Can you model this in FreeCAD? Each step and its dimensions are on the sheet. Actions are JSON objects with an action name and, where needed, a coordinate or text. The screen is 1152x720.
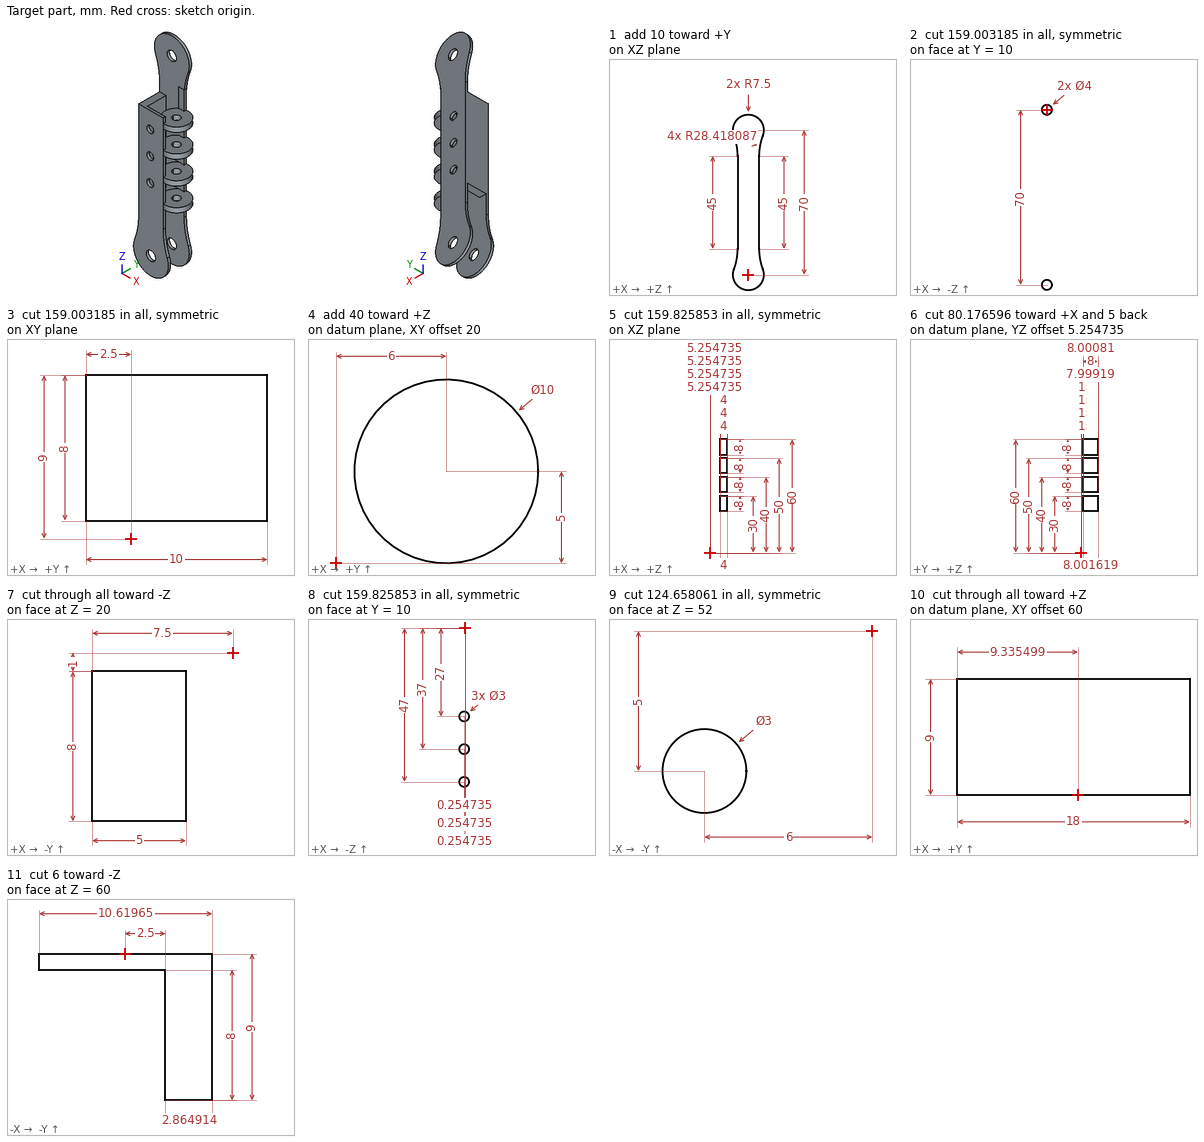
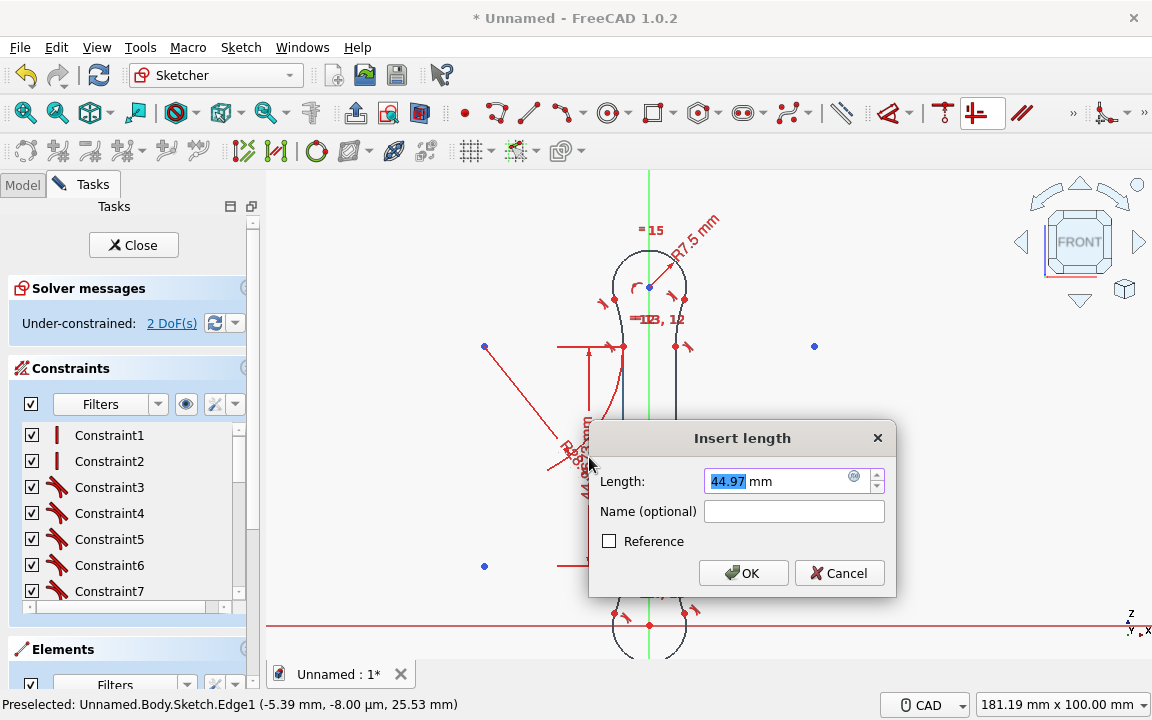
{"action": "type", "text": "45"}
{"action": "key", "text": "Return"}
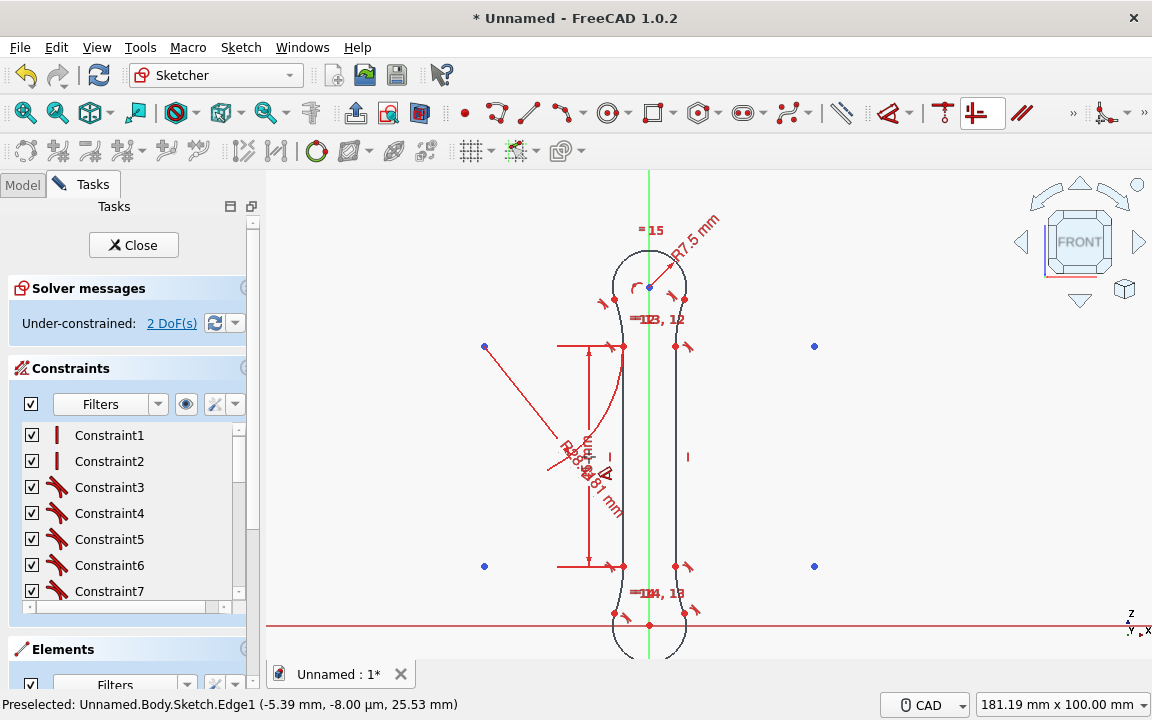
{"action": "left_click", "coordinate": [676, 412]}
{"action": "left_click", "coordinate": [710, 457]}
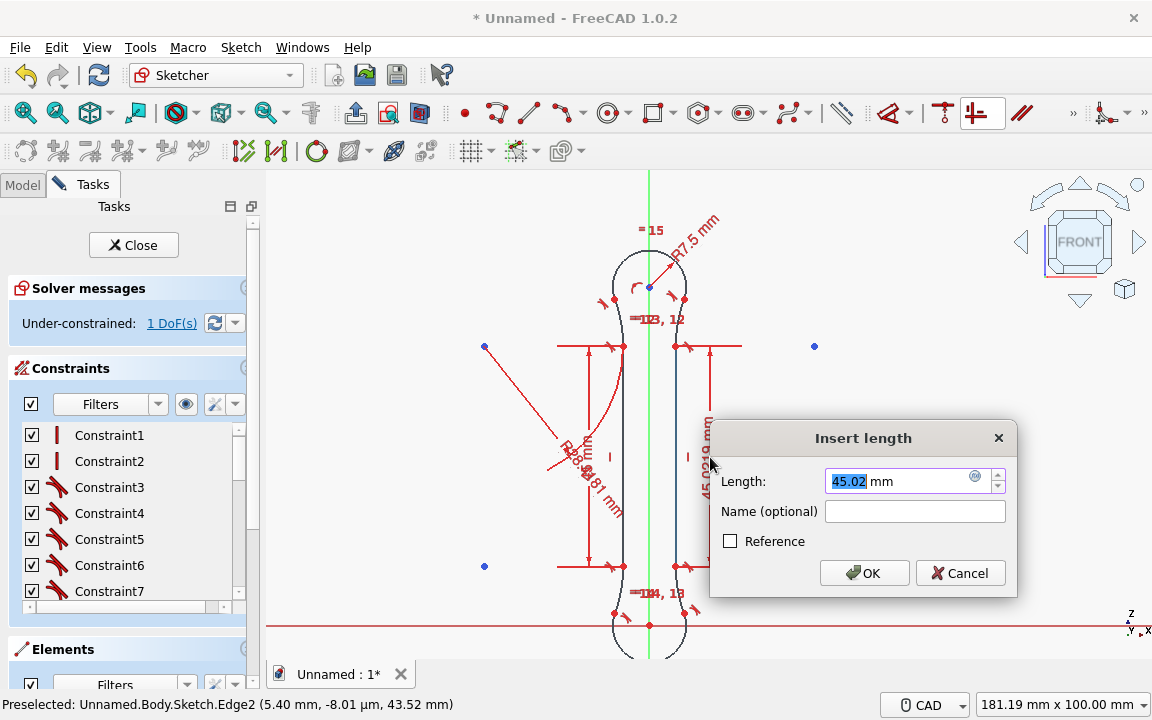
{"action": "type", "text": "45"}
{"action": "key", "text": "Return"}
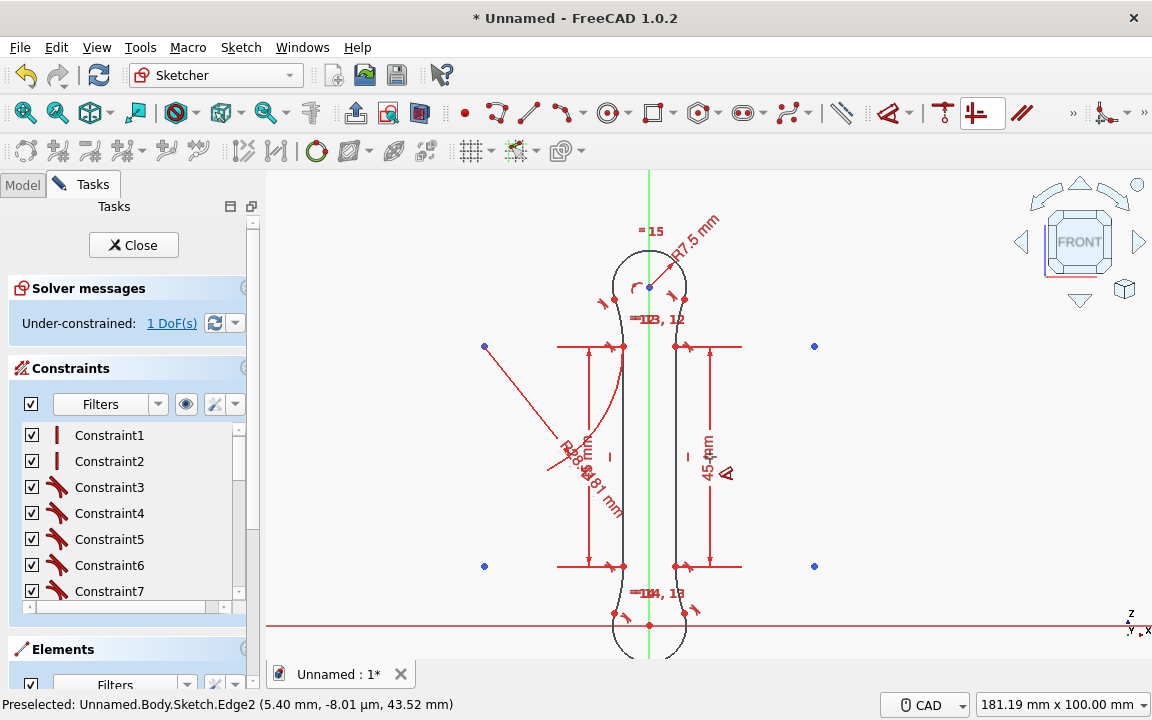
{"action": "left_click", "coordinate": [649, 287]}
{"action": "left_click", "coordinate": [707, 379]}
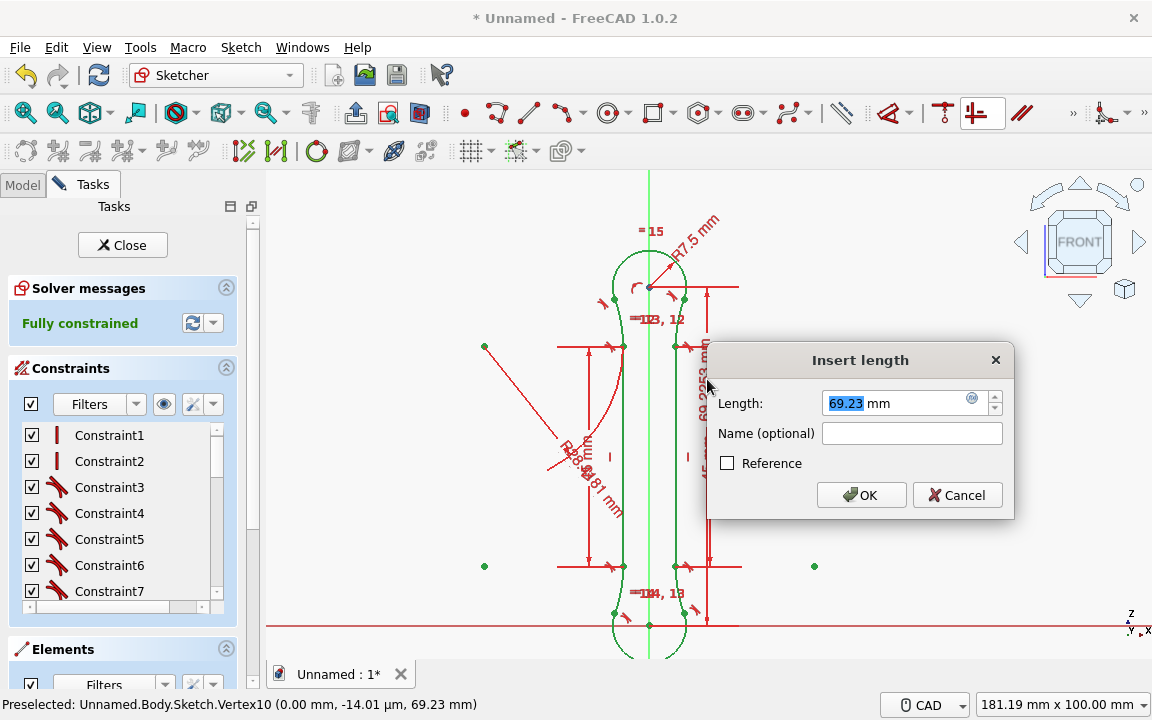
{"action": "type", "text": "70"}
{"action": "key", "text": "Return"}
{"action": "key", "text": "Escape"}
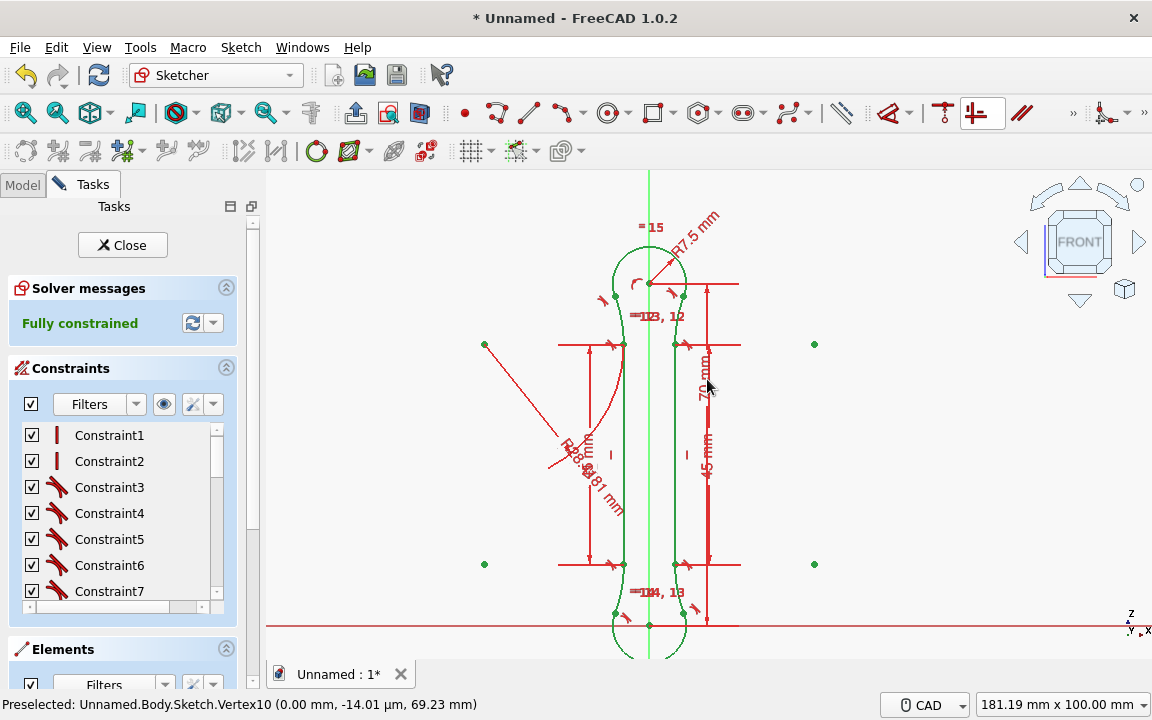
{"action": "left_click", "coordinate": [123, 245]}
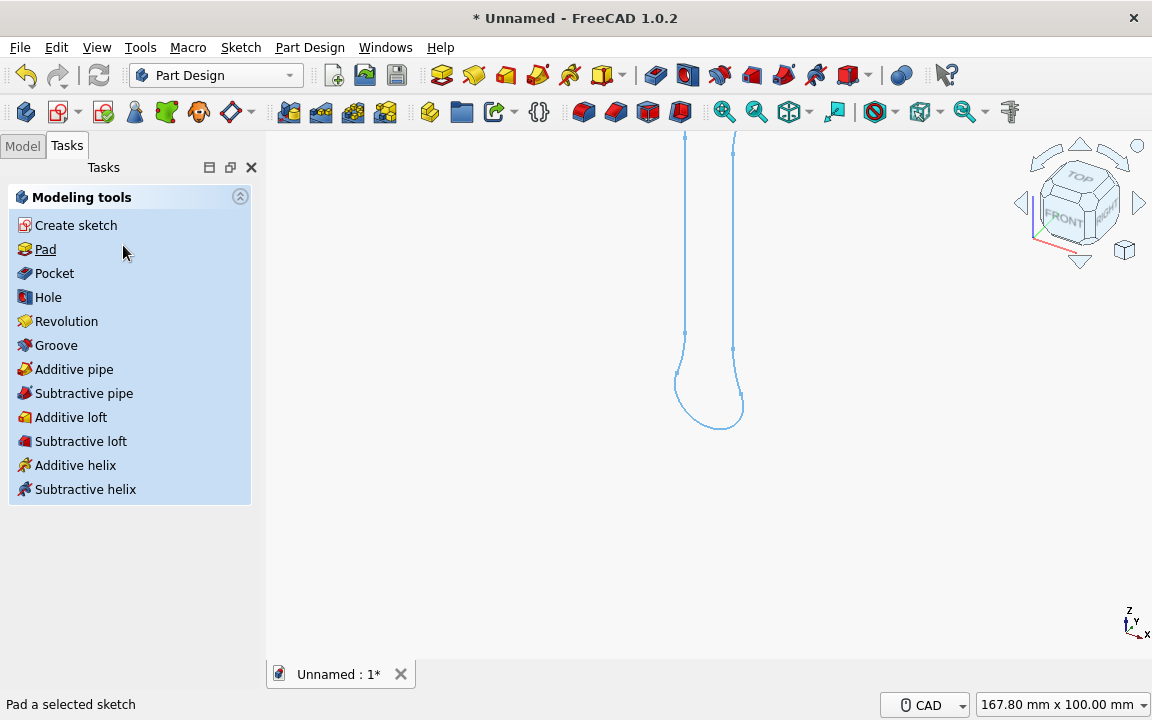
{"action": "left_click", "coordinate": [442, 76]}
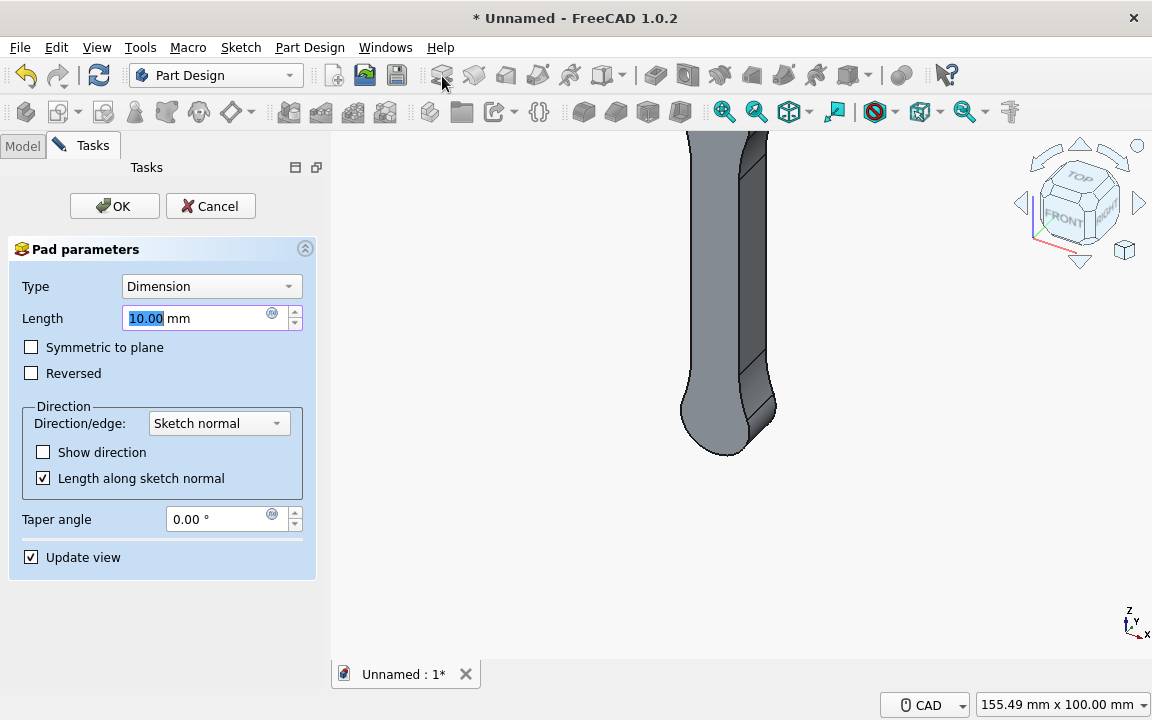
{"action": "type", "text": "10"}
{"action": "key", "text": "Tab"}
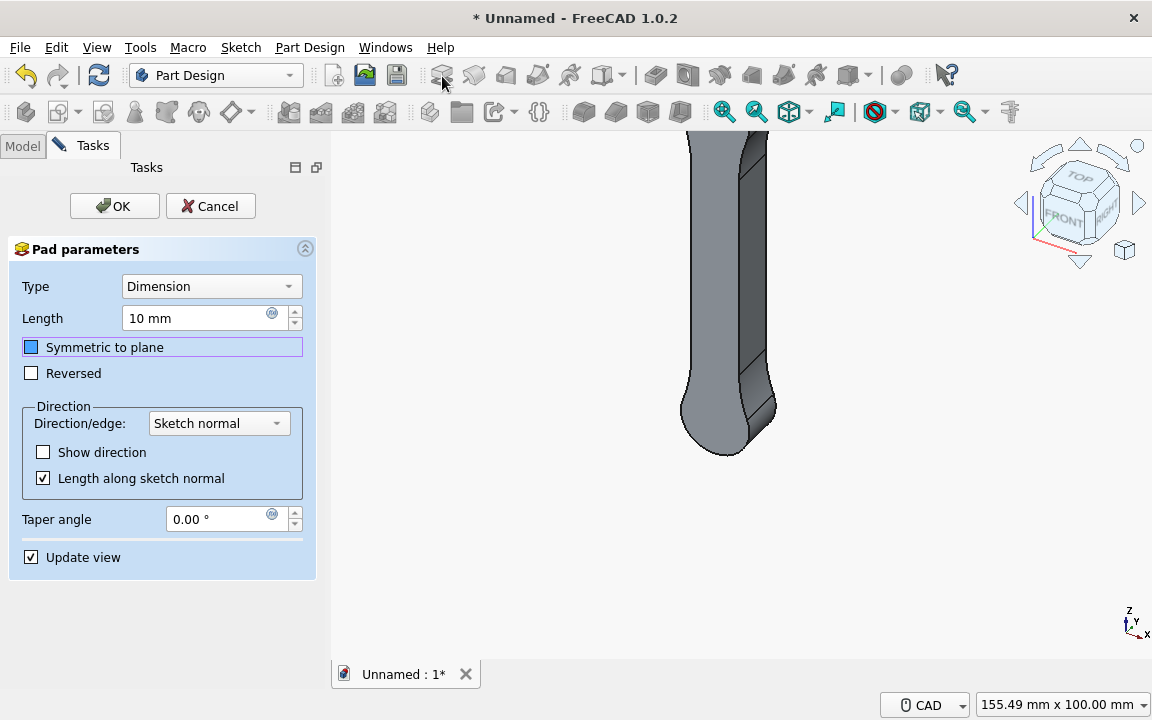
{"action": "left_click", "coordinate": [30, 373]}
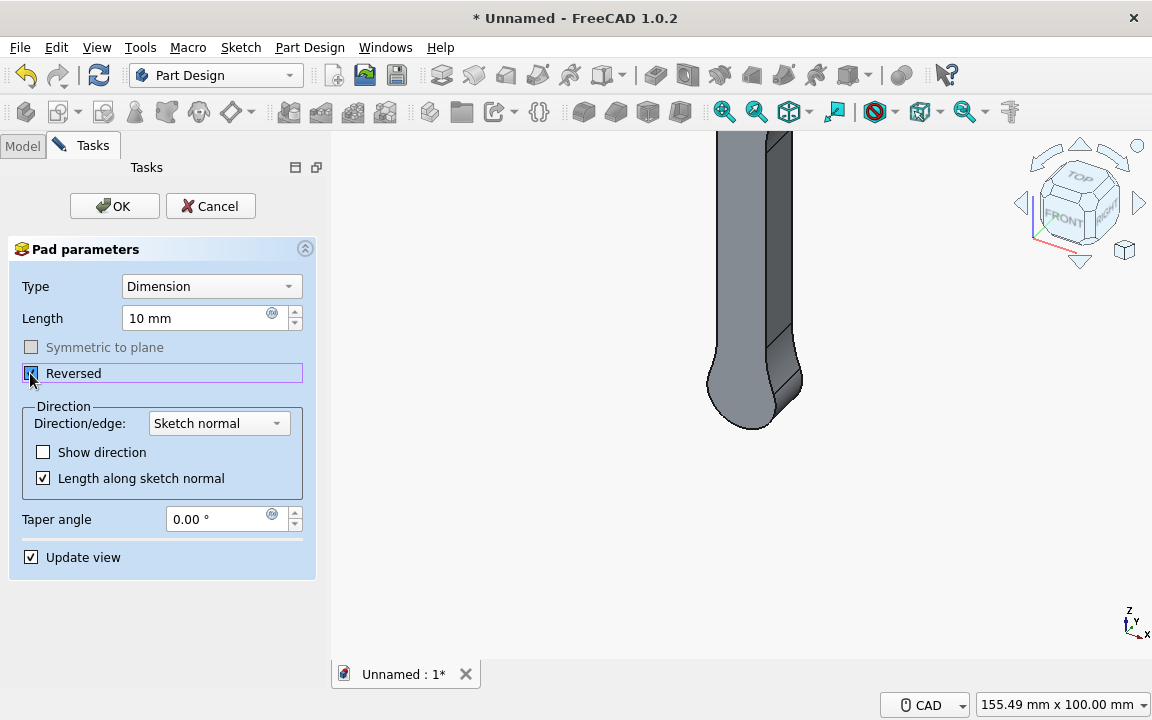
{"action": "left_click", "coordinate": [115, 206]}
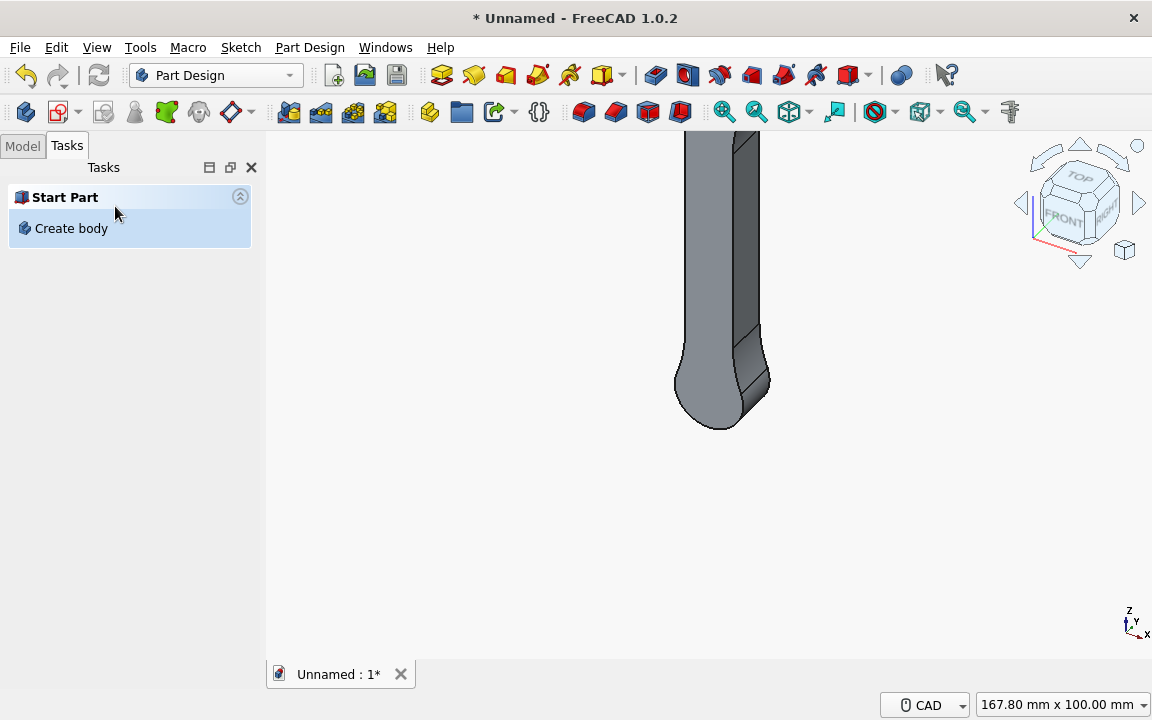
{"action": "left_click", "coordinate": [726, 112]}